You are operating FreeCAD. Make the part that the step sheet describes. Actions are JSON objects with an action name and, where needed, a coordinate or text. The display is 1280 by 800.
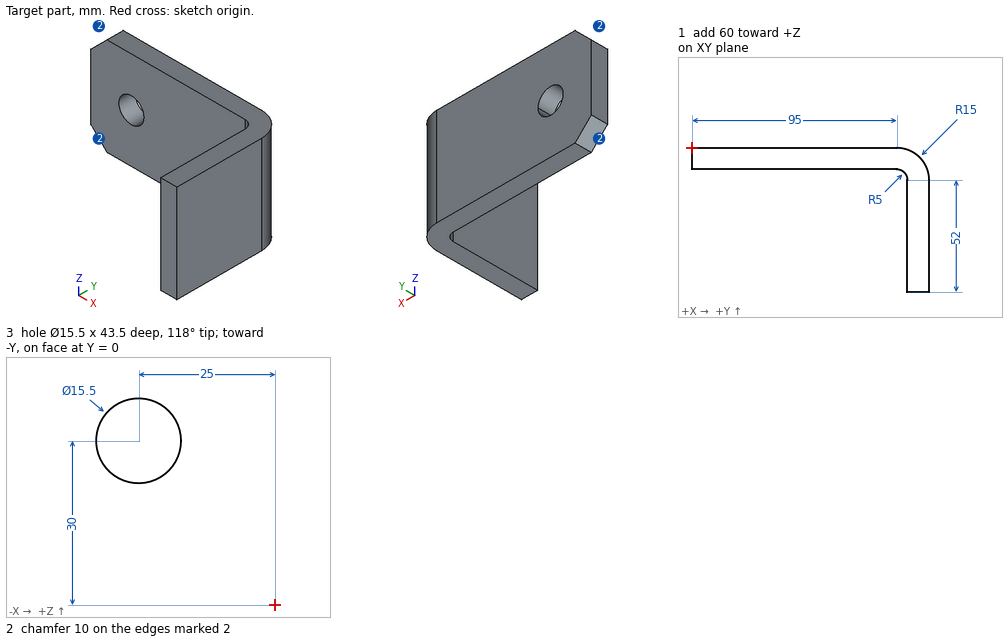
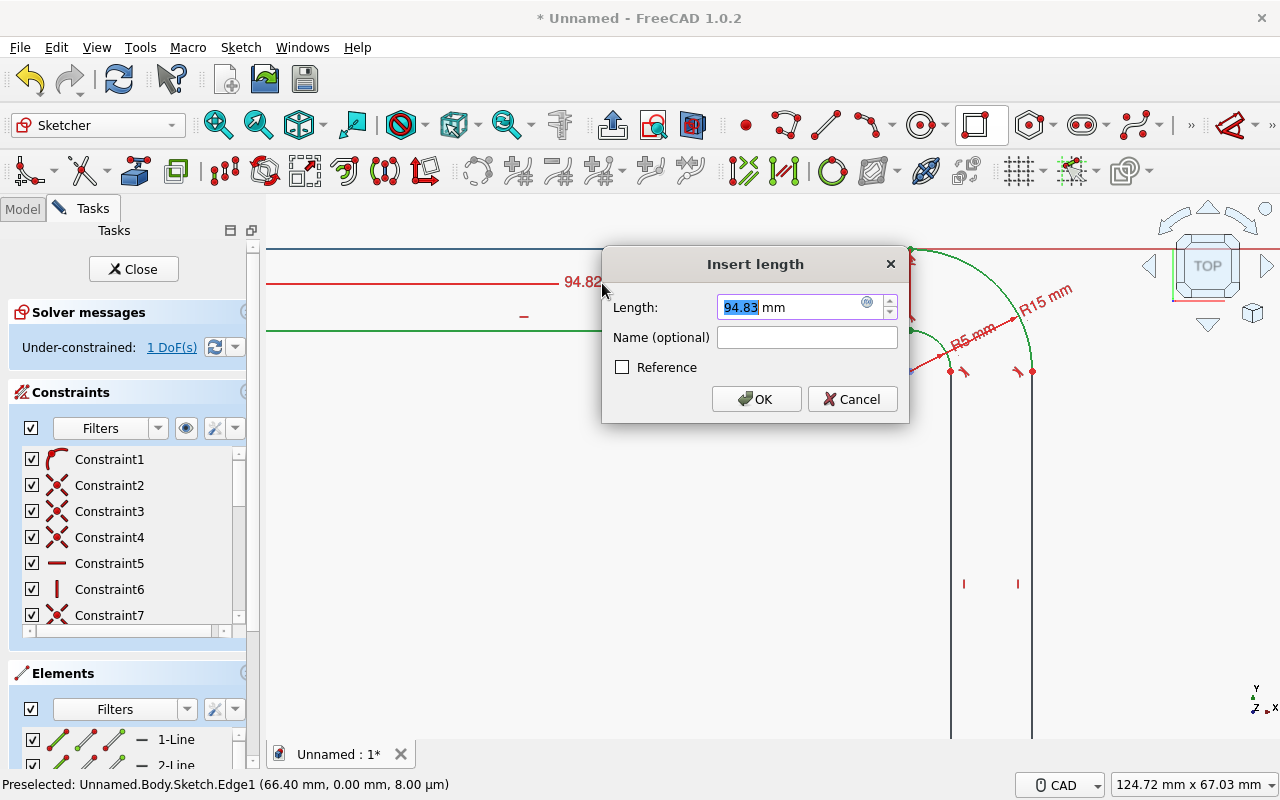
{"action": "type", "text": "95"}
{"action": "key", "text": "Return"}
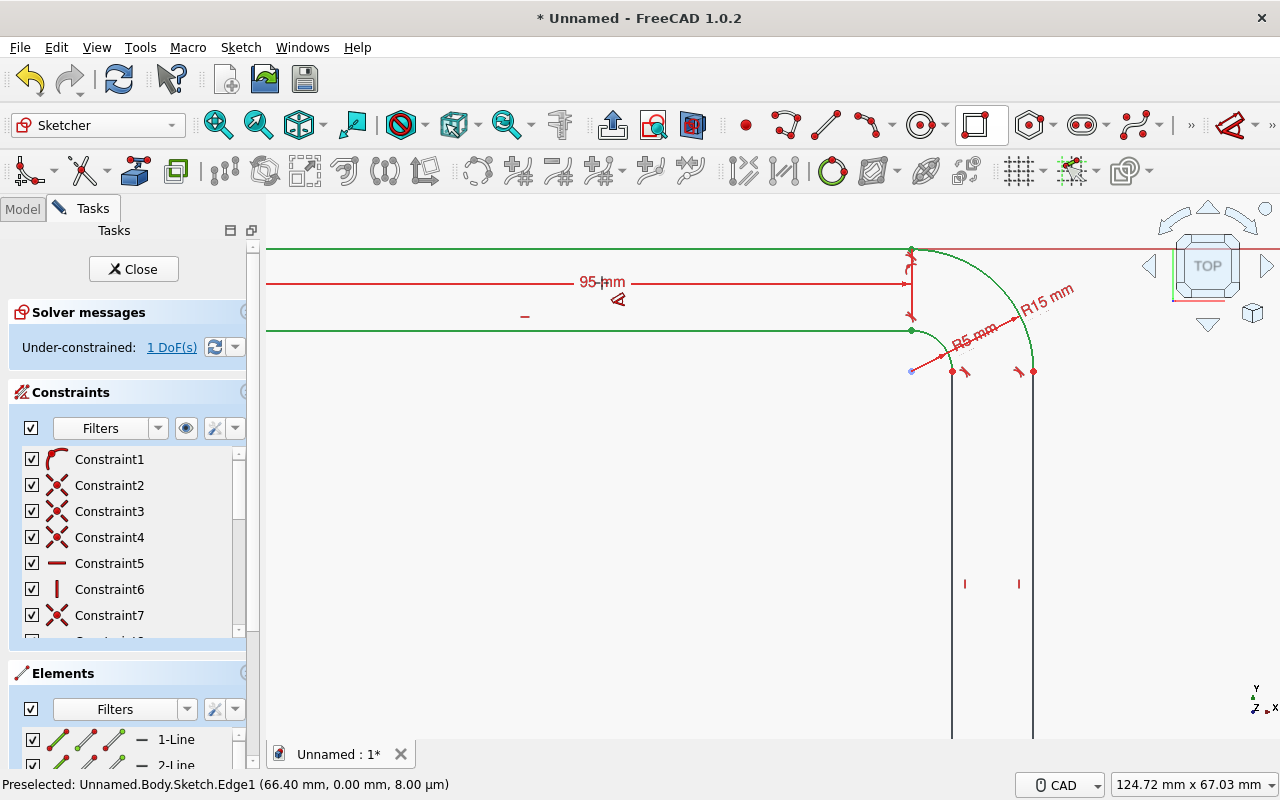
{"action": "left_click", "coordinate": [952, 499]}
{"action": "left_click", "coordinate": [986, 541]}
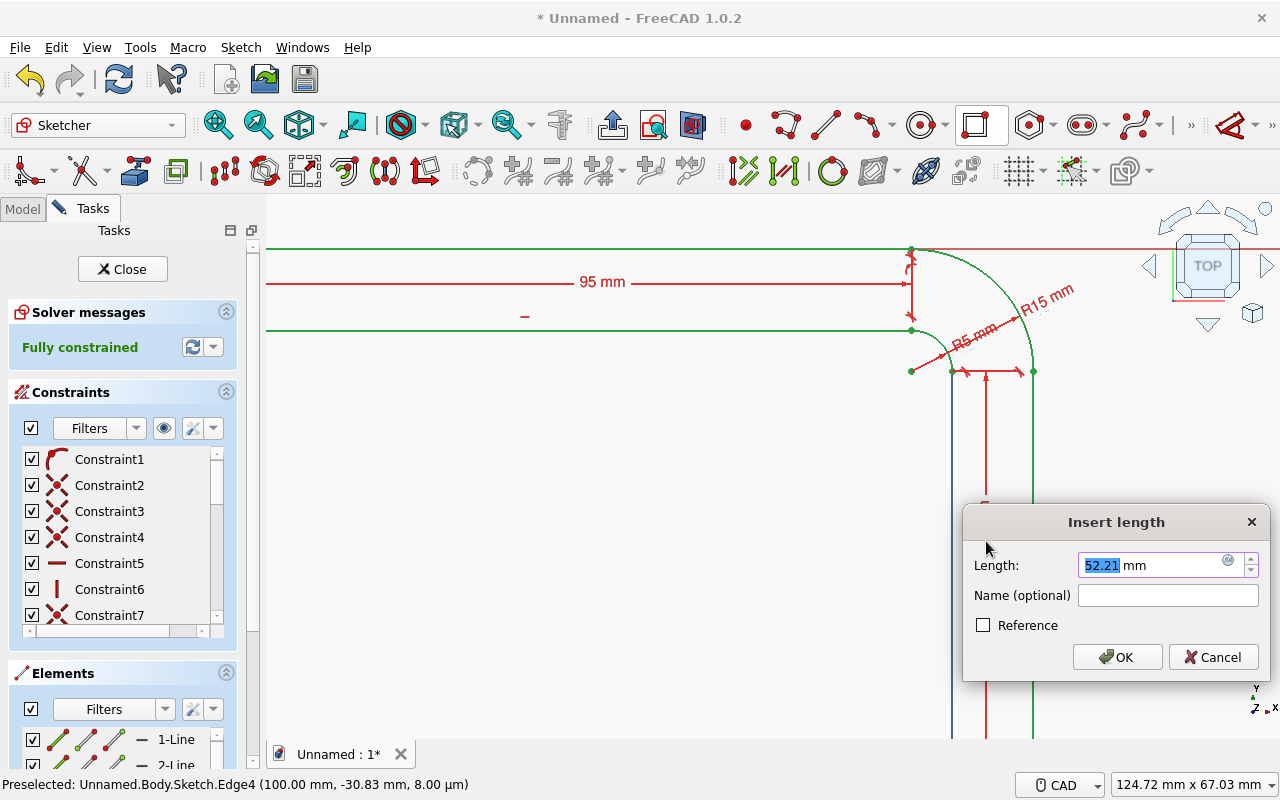
{"action": "type", "text": "52"}
{"action": "key", "text": "Return"}
{"action": "key", "text": "Escape"}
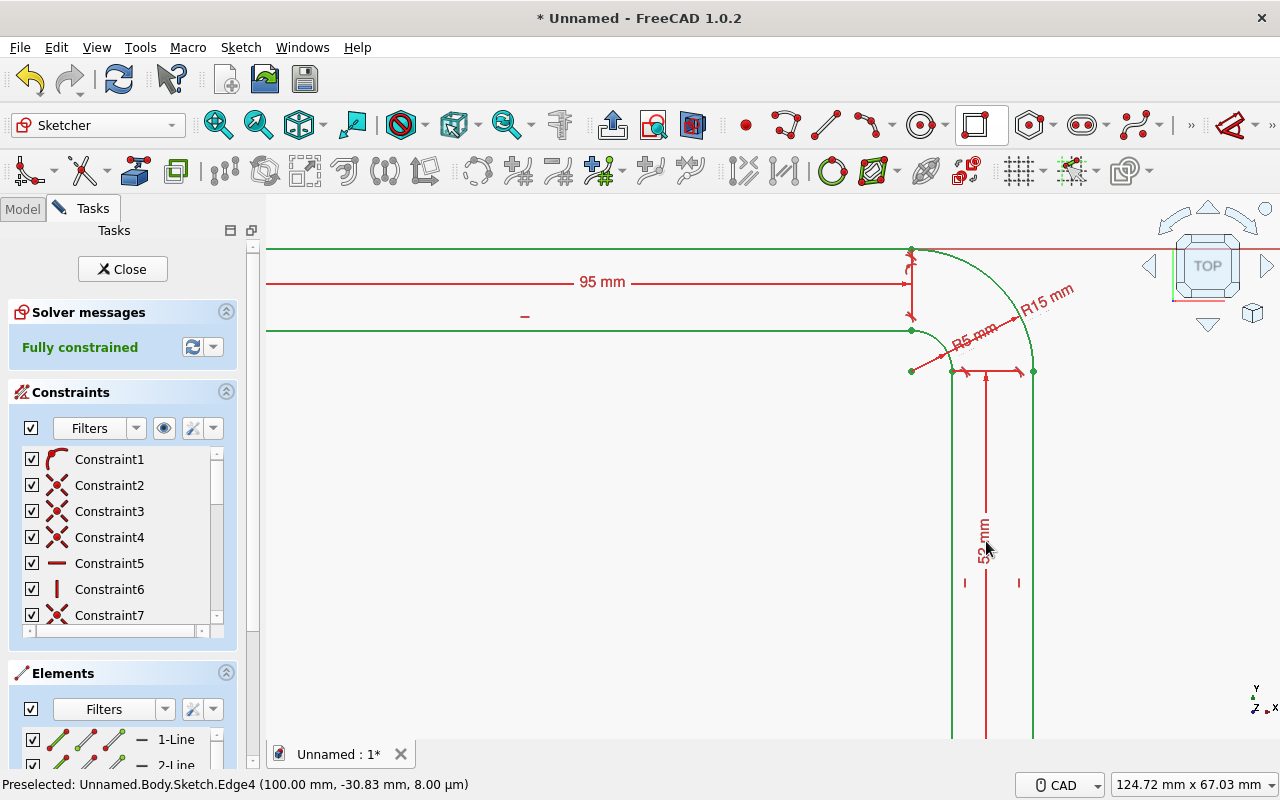
{"action": "left_click", "coordinate": [123, 269]}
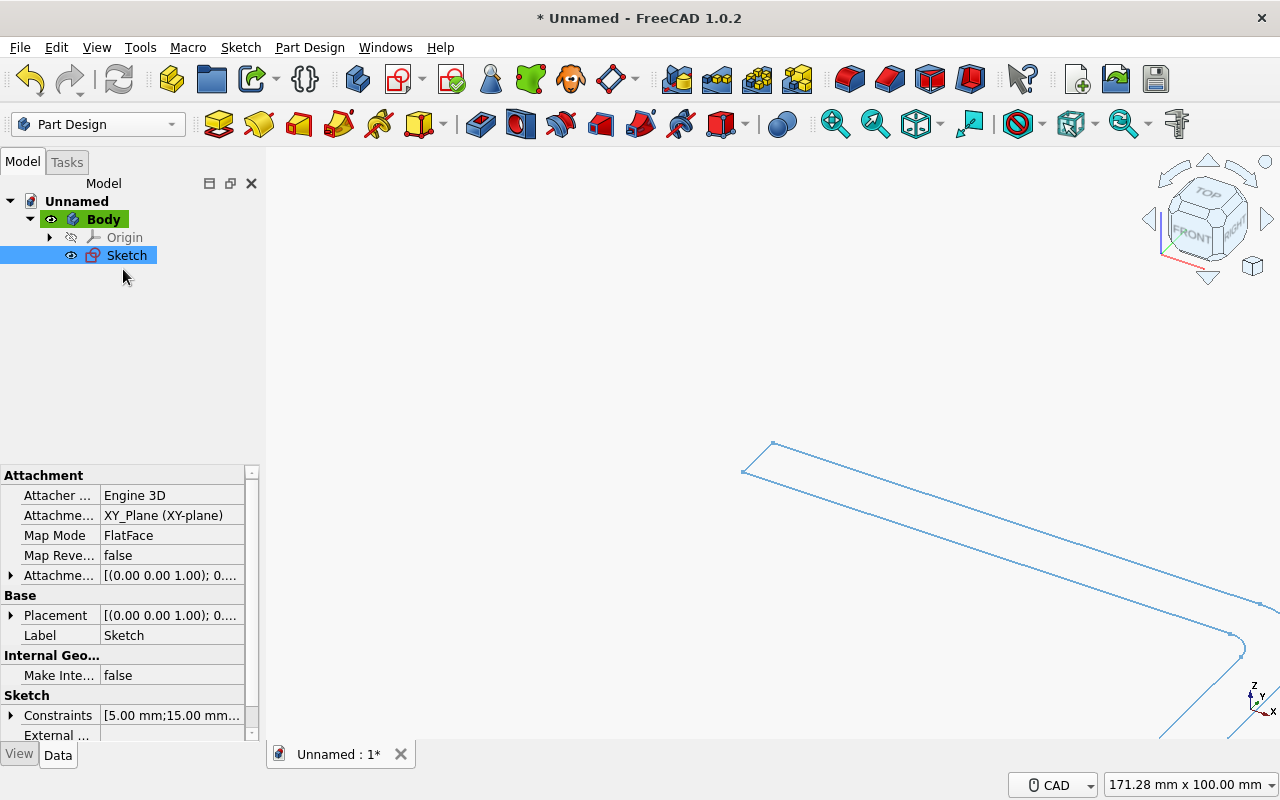
{"action": "left_click", "coordinate": [220, 124]}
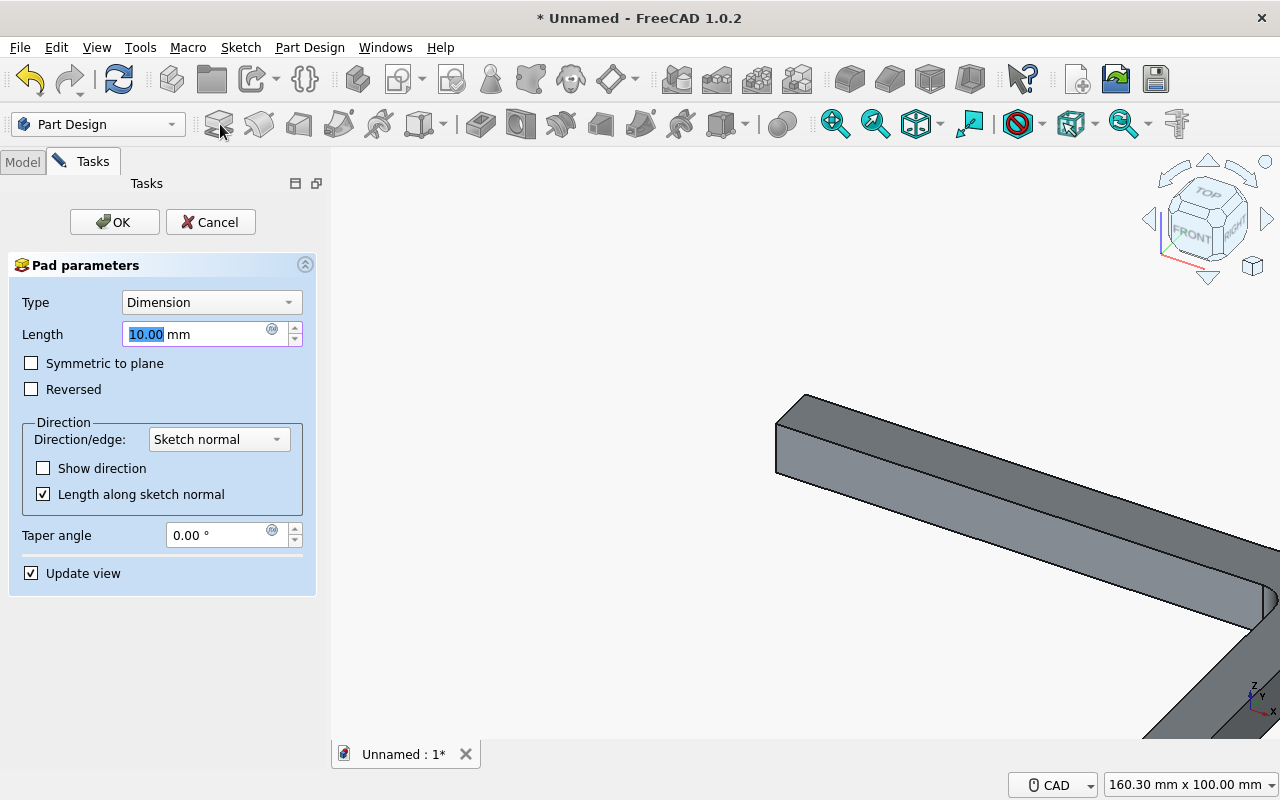
{"action": "type", "text": "60"}
{"action": "key", "text": "Tab"}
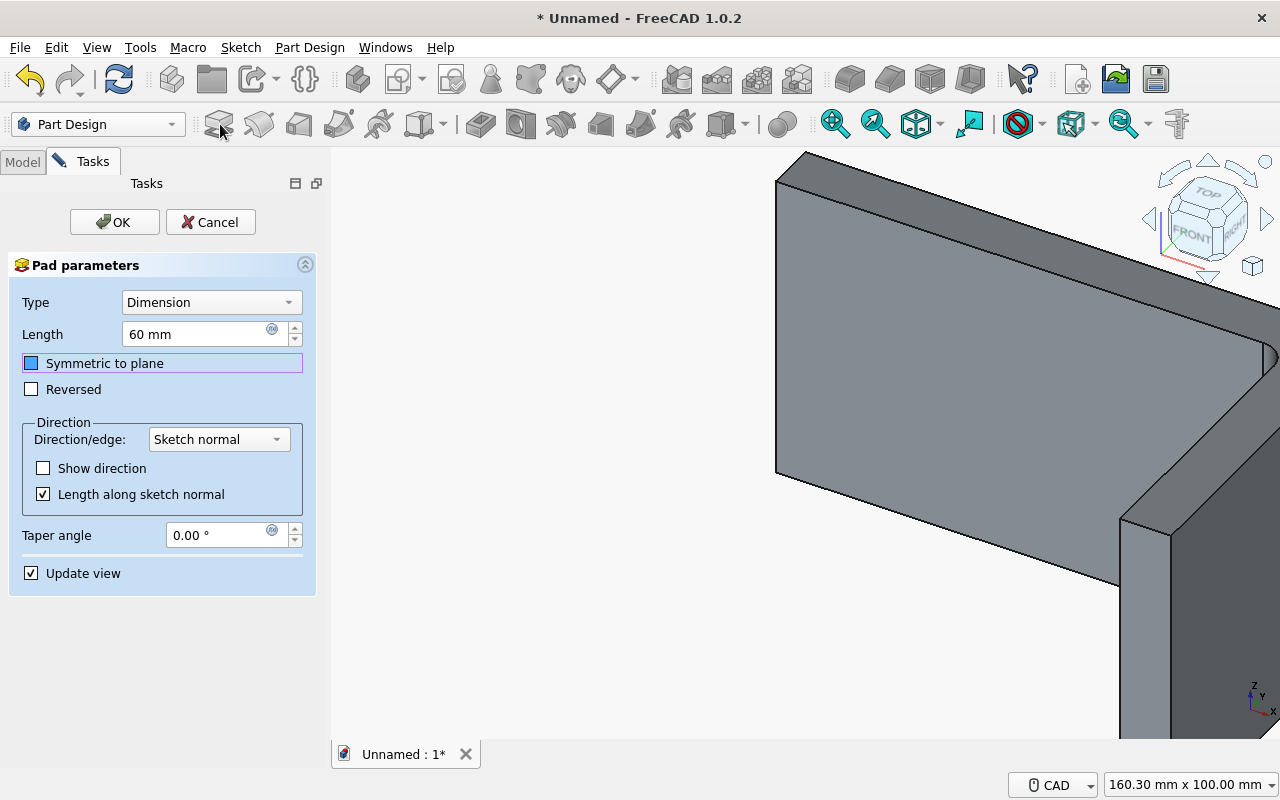
{"action": "left_click", "coordinate": [115, 222]}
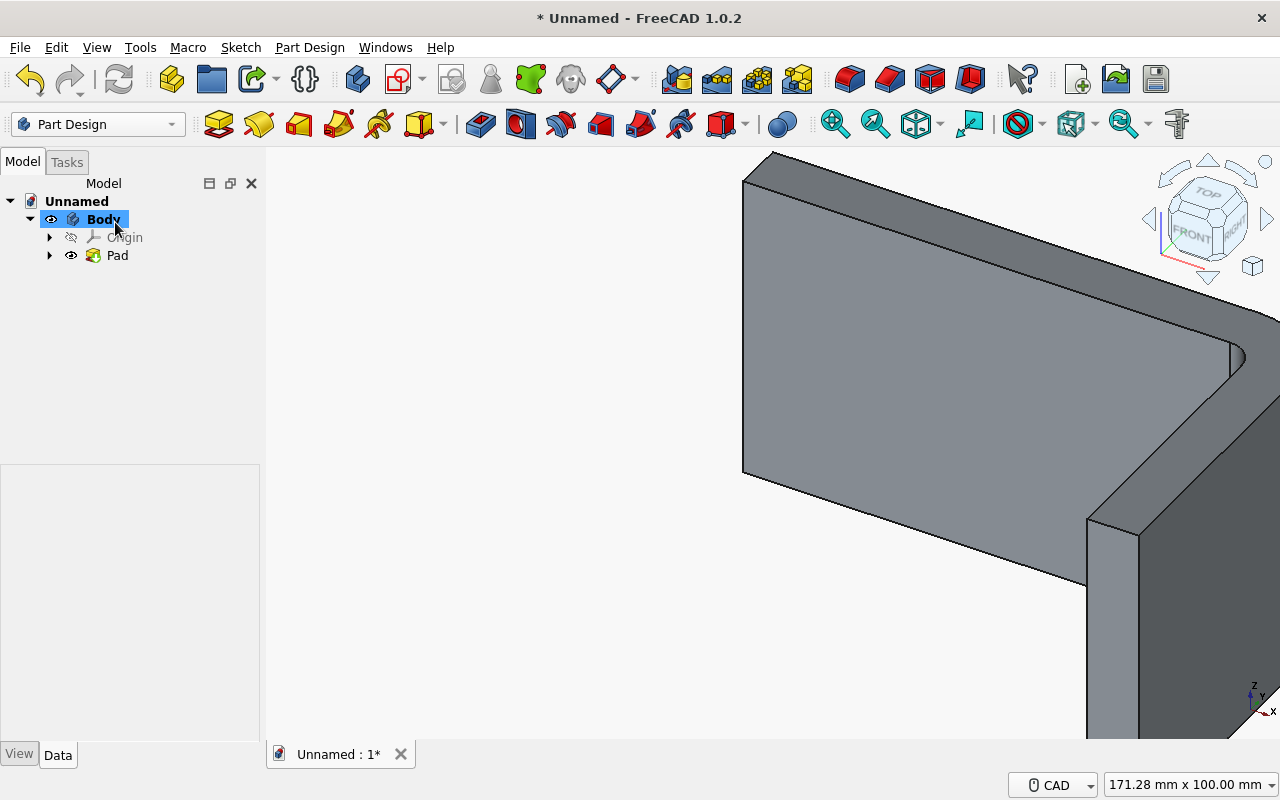
{"action": "left_click", "coordinate": [836, 124]}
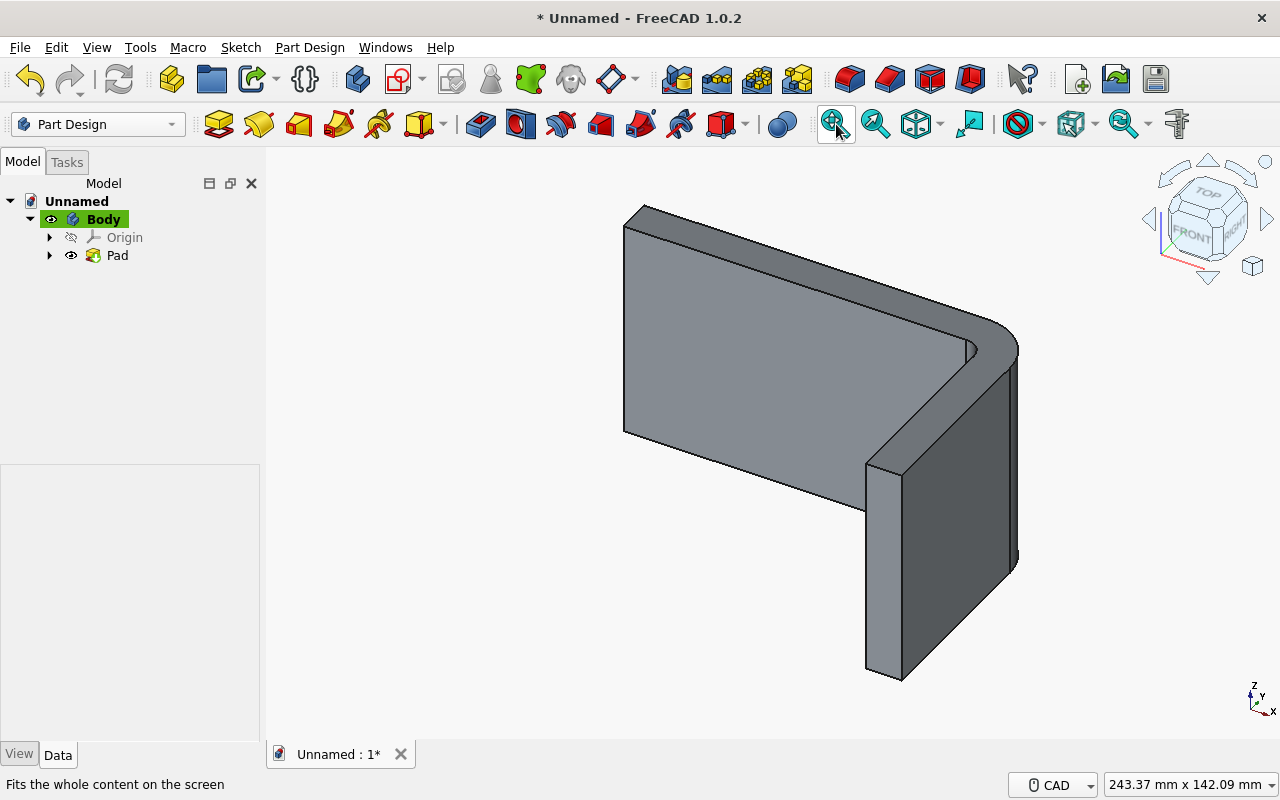
{"action": "key", "text": "0"}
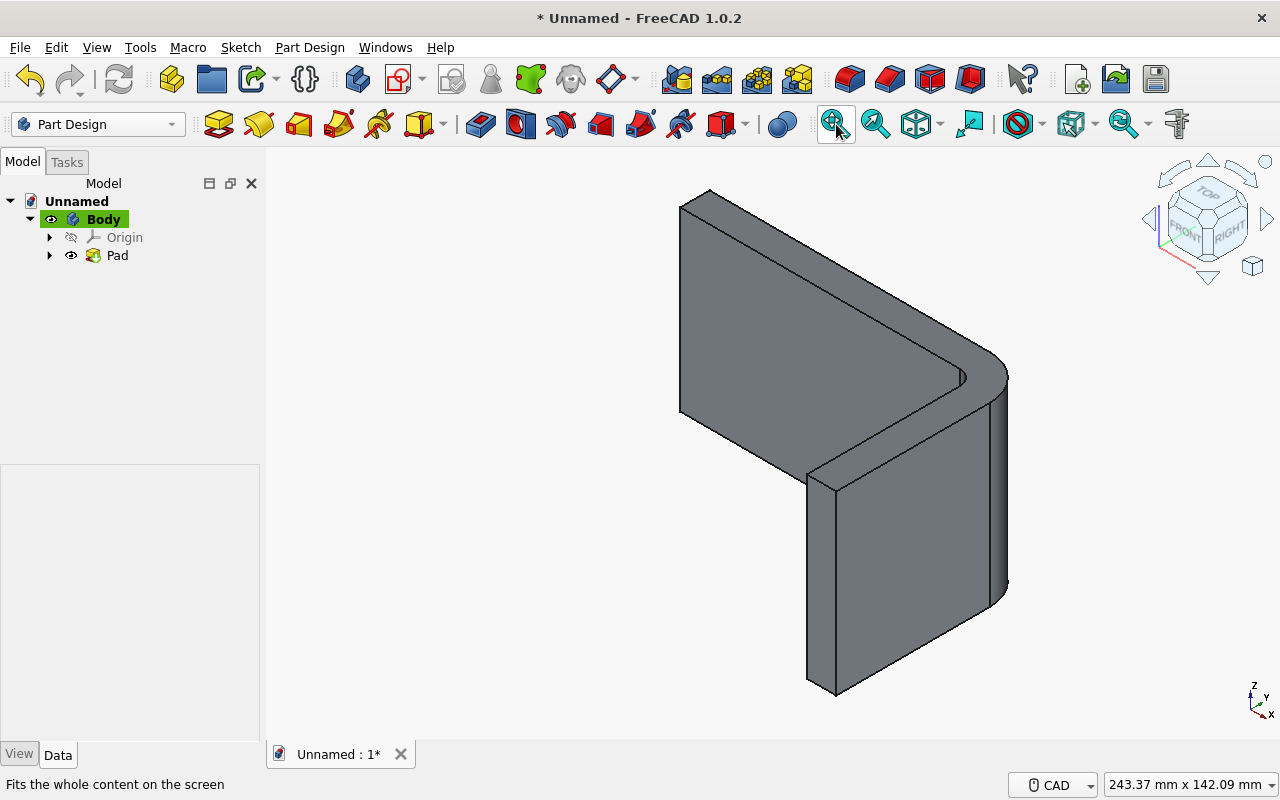
{"action": "key", "text": "2"}